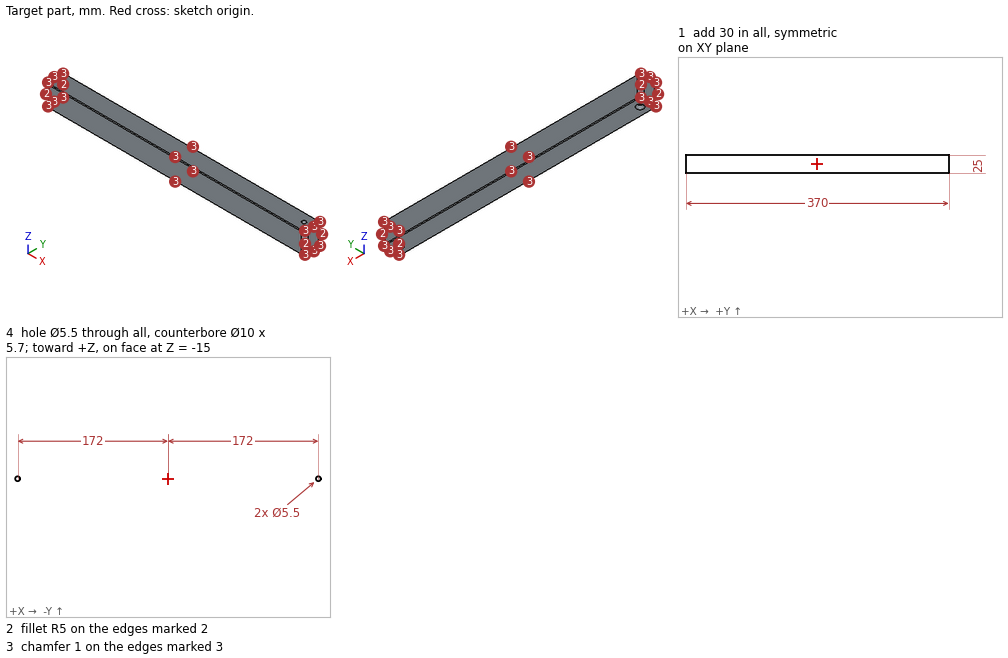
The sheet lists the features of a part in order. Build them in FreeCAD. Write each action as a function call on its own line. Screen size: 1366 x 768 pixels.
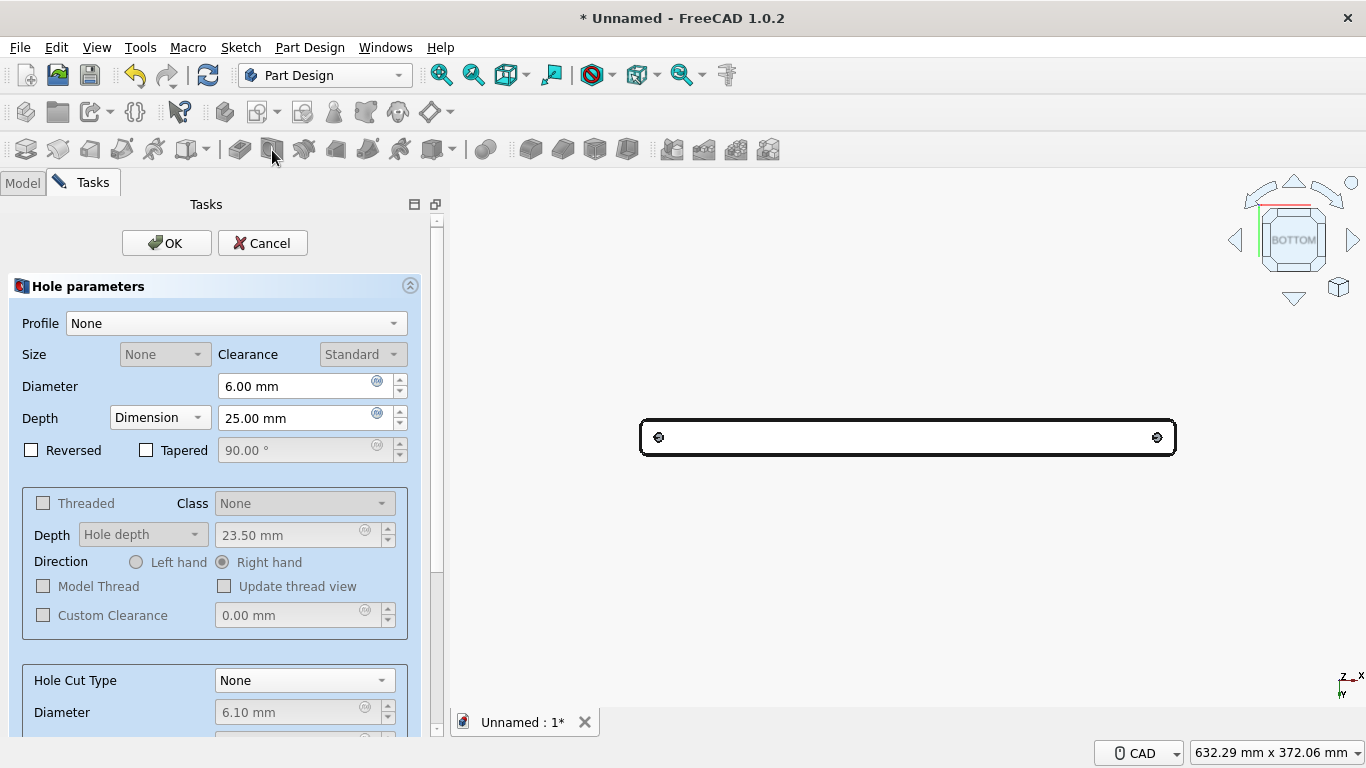
triple_click(305, 386)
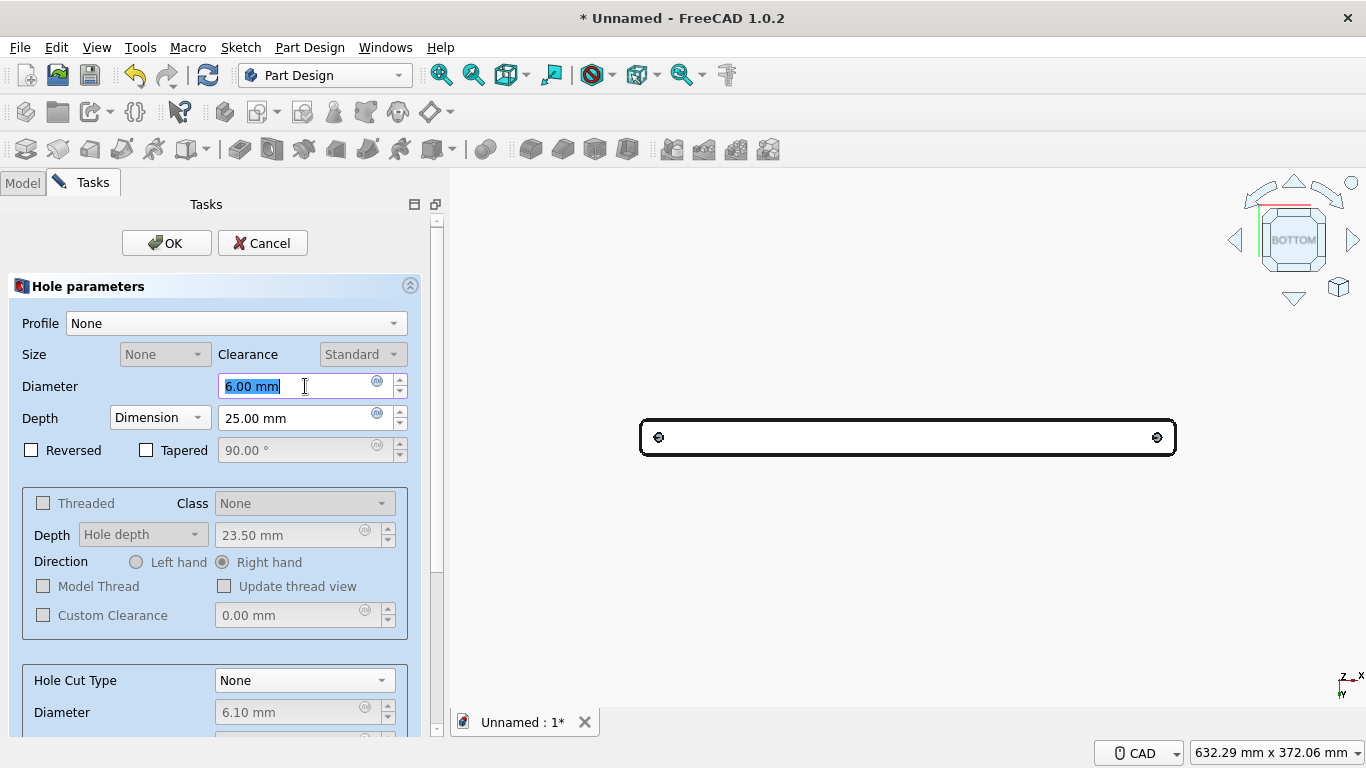
text(5.5)
key(Tab)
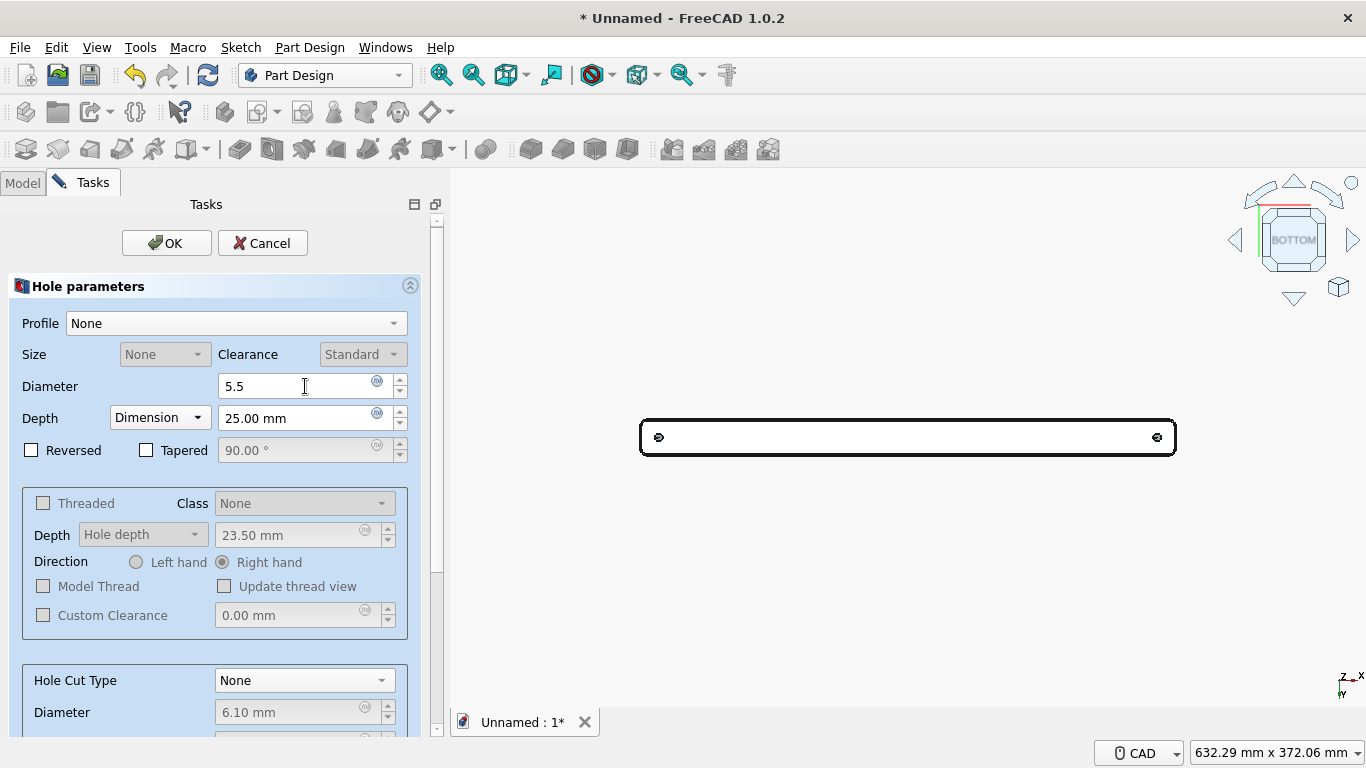
click(161, 418)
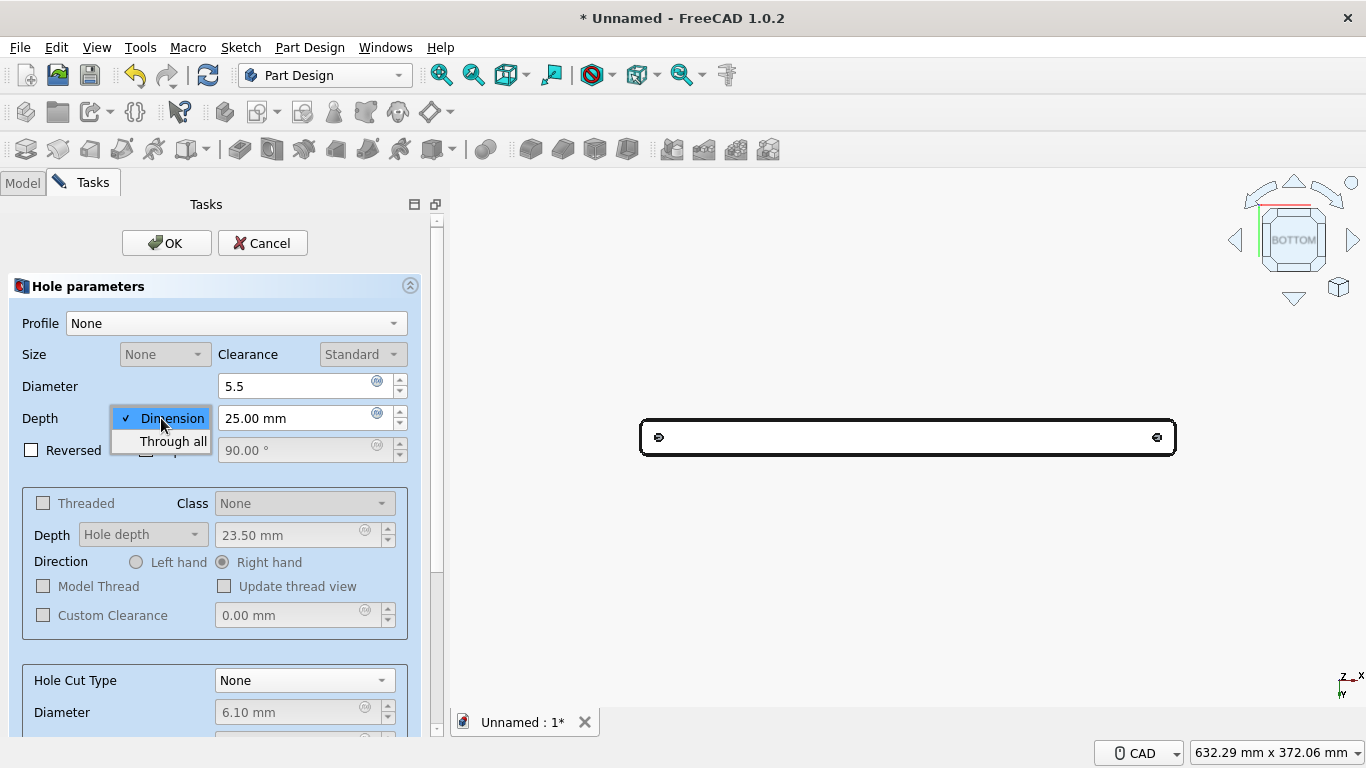
click(160, 442)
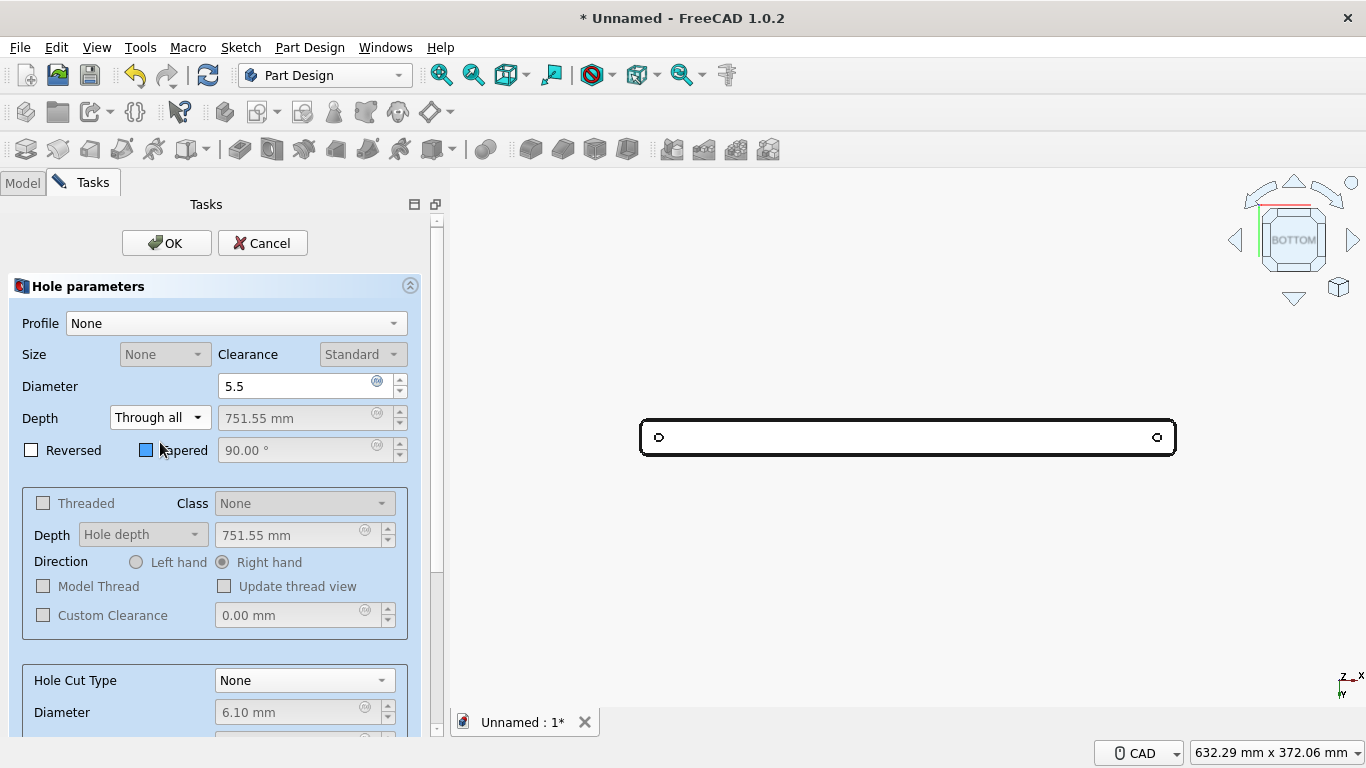
click(306, 680)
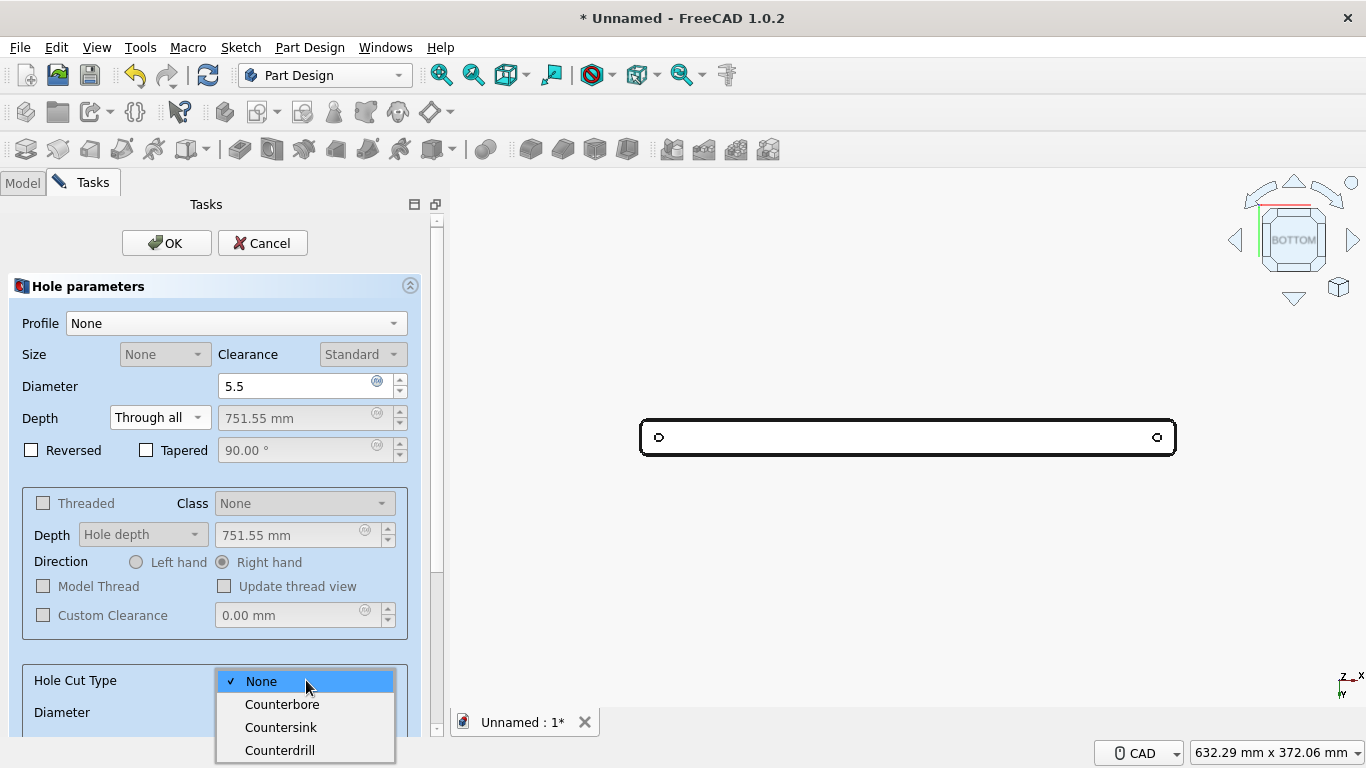
click(304, 704)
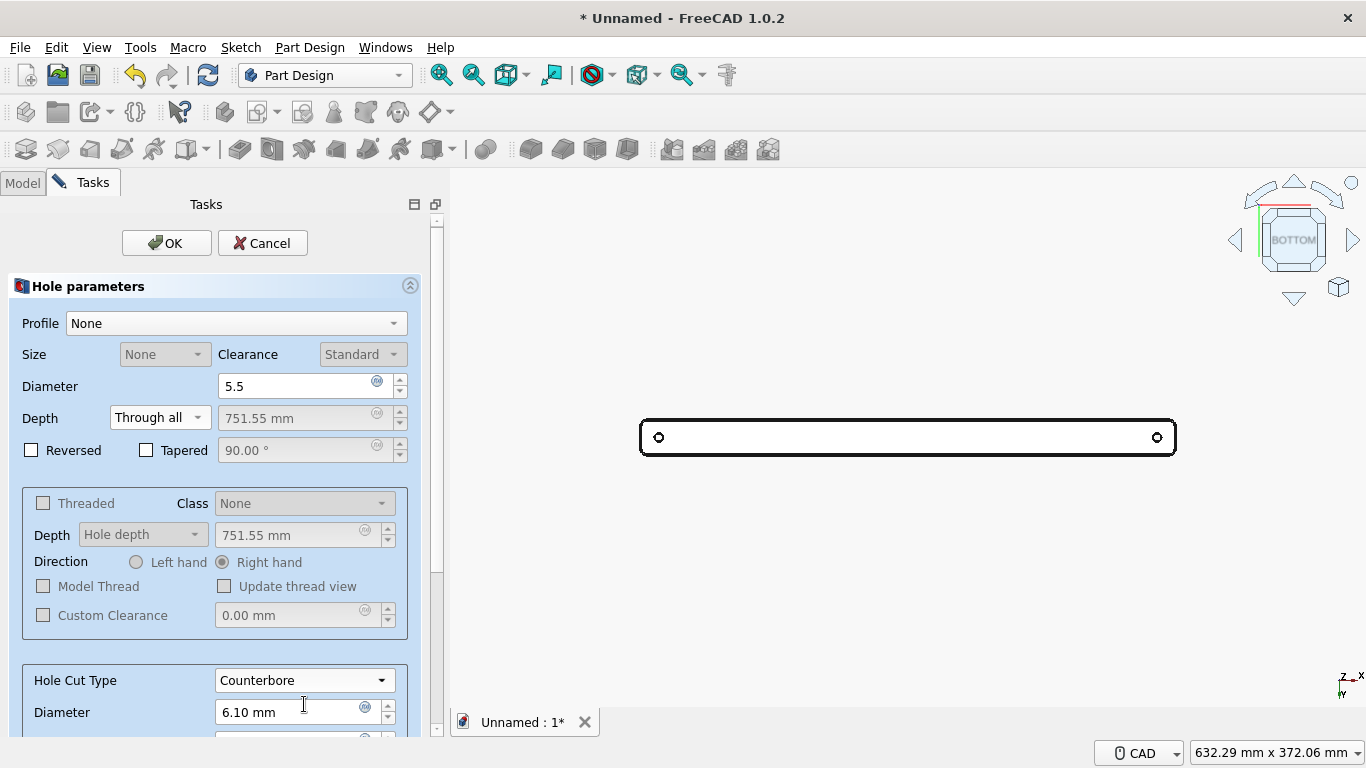
triple_click(298, 712)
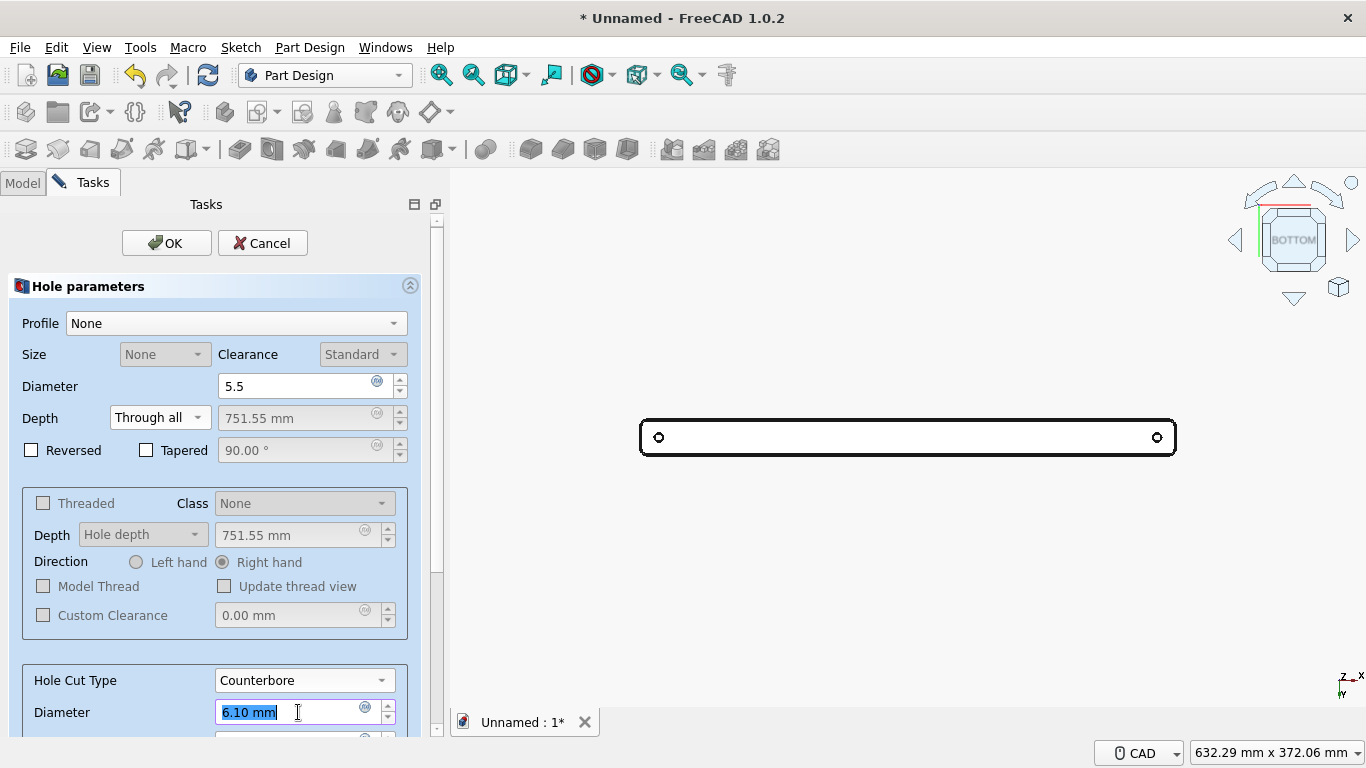
text(10)
key(Tab)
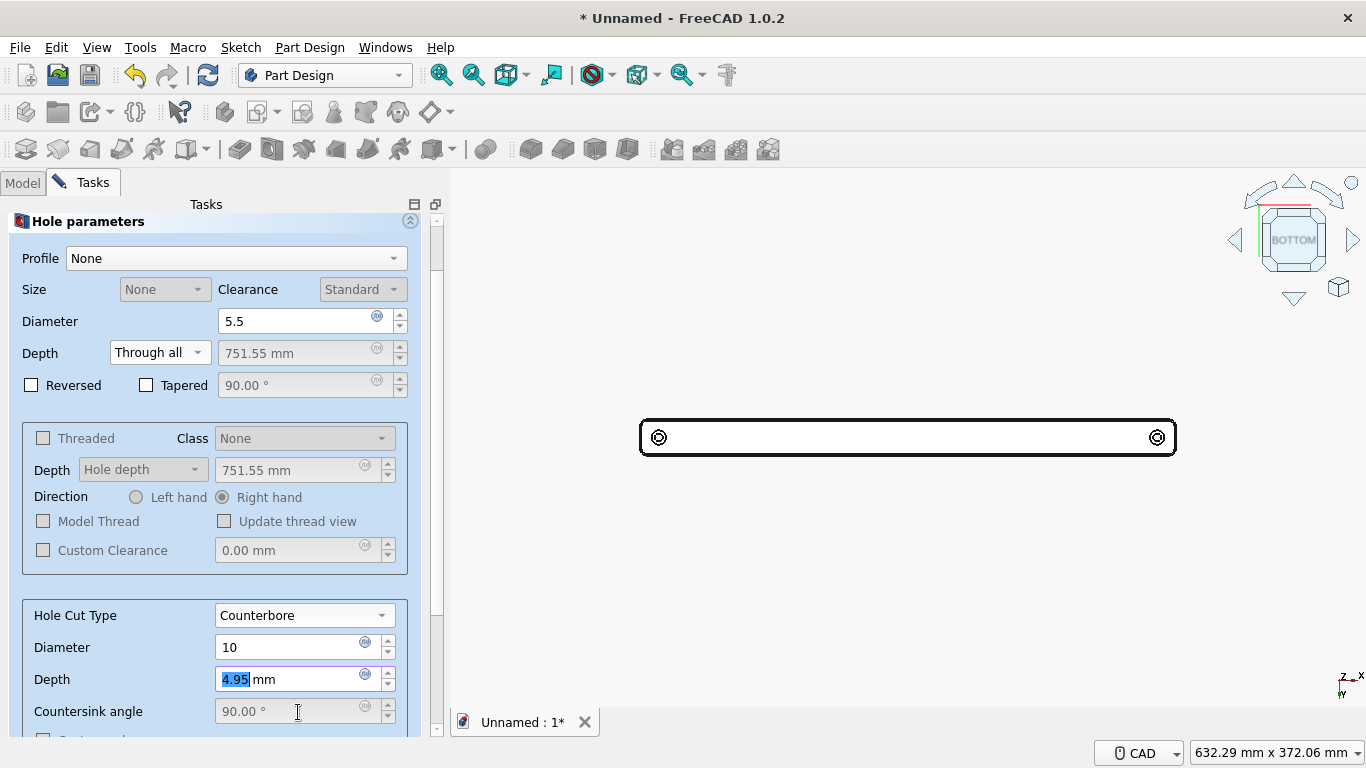
text(5.7)
key(Tab)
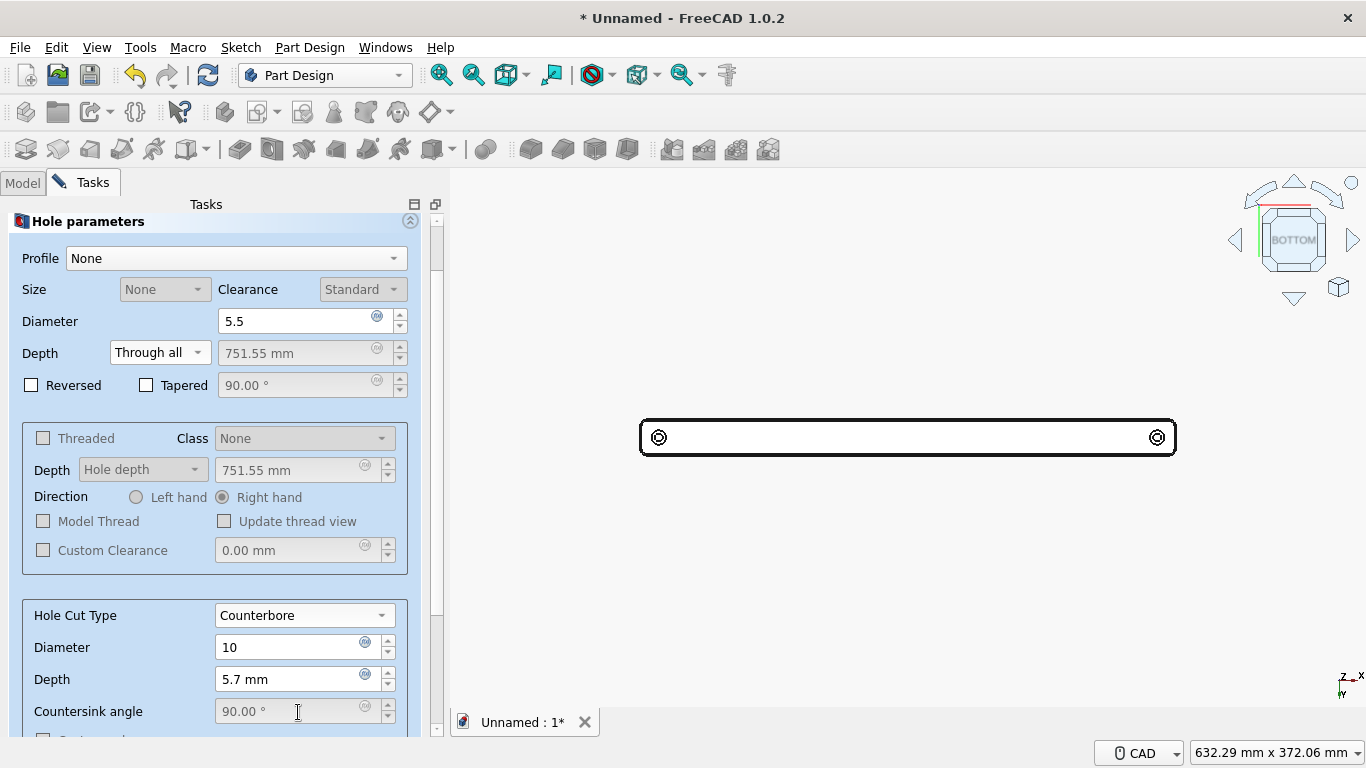
scroll(437, 475, up, 2)